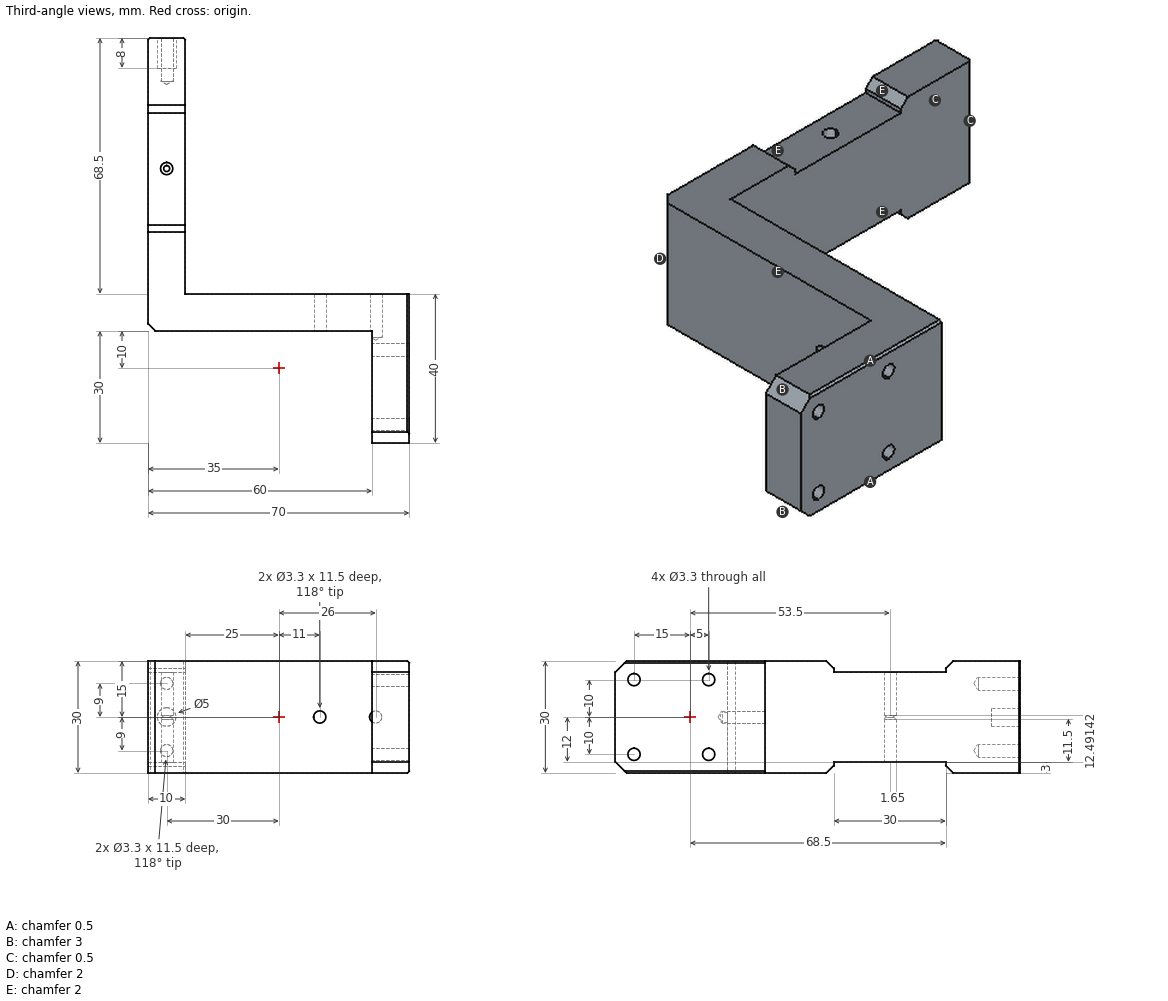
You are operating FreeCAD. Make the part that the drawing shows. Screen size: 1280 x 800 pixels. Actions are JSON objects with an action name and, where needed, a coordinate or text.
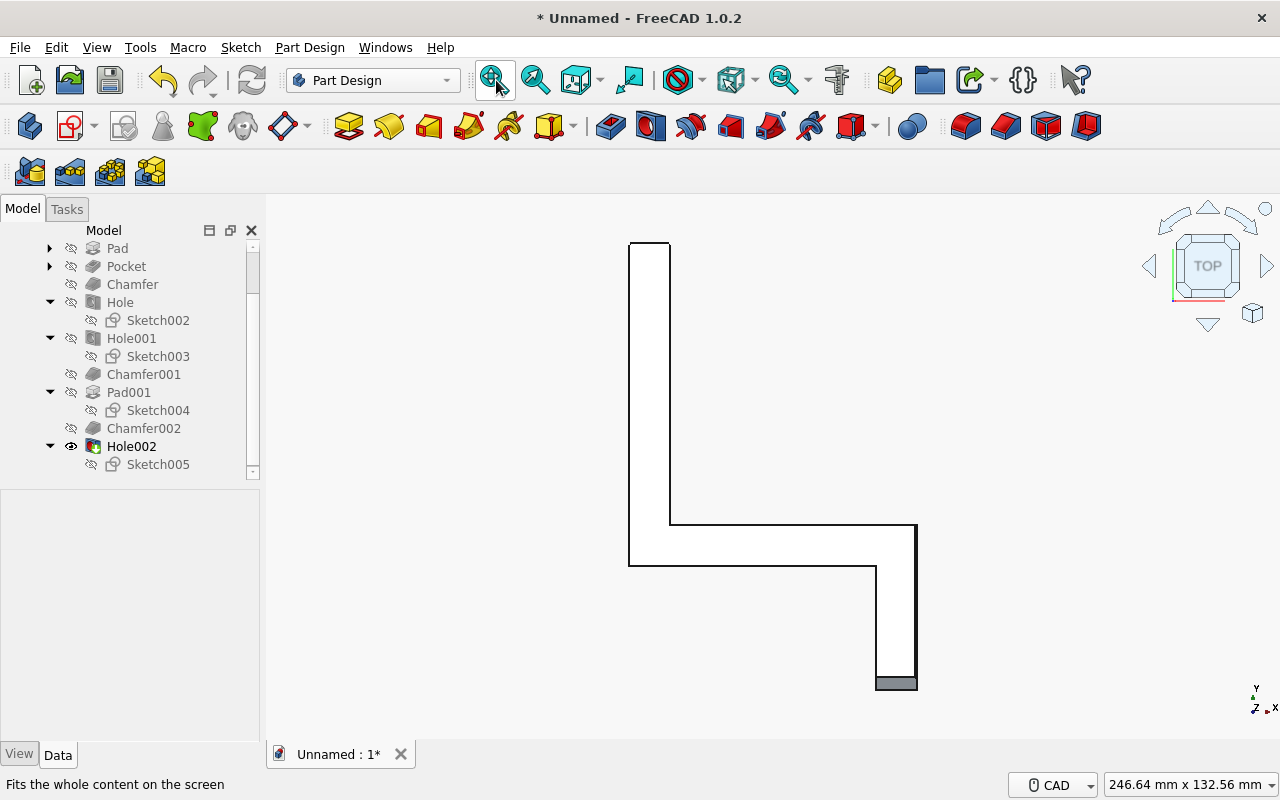
{"action": "key", "text": "1"}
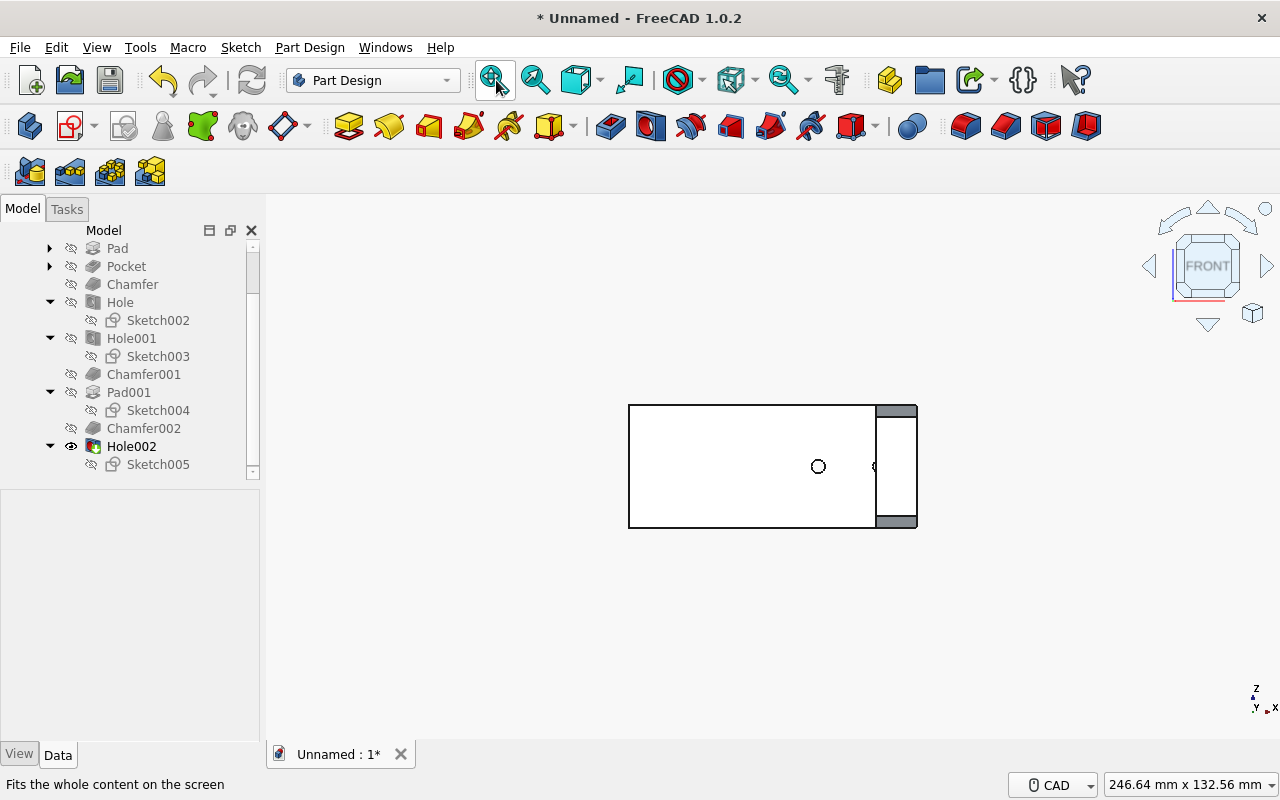
{"action": "left_click", "coordinate": [496, 80]}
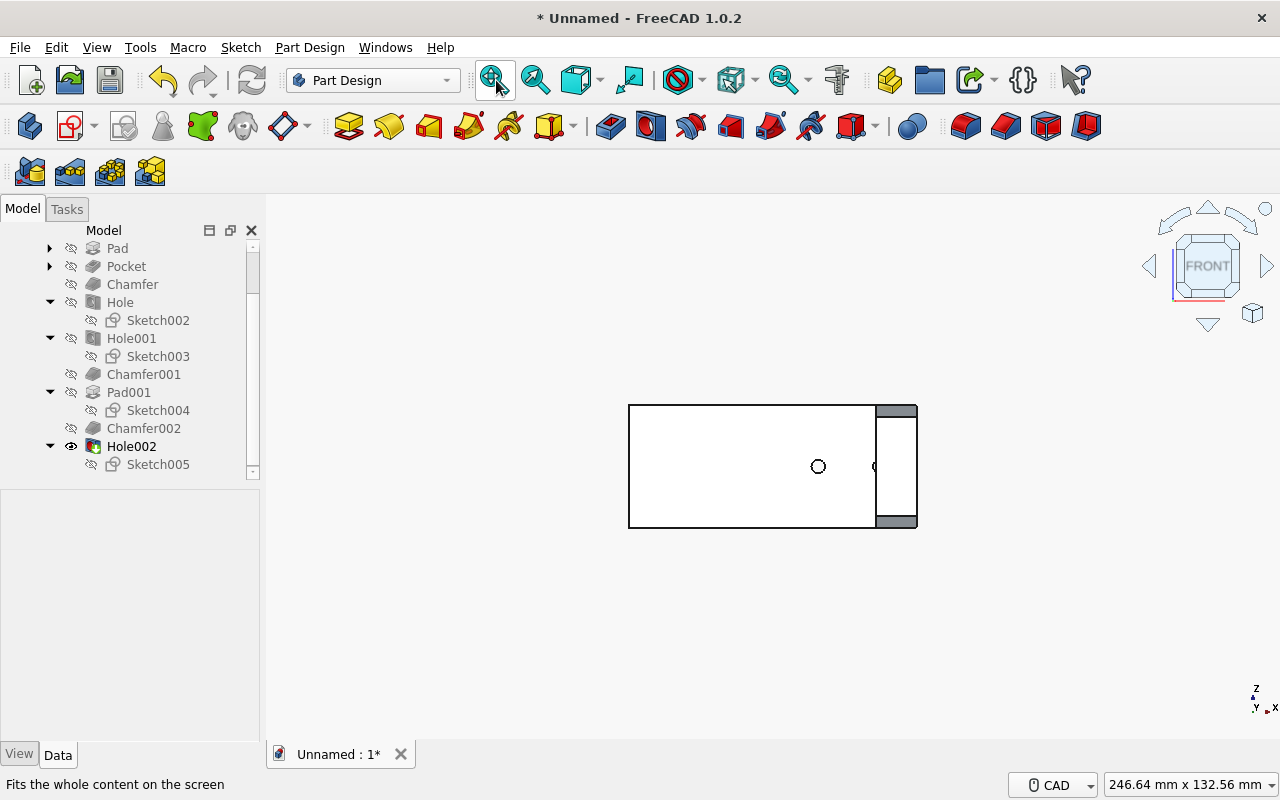
{"action": "left_click", "coordinate": [629, 466]}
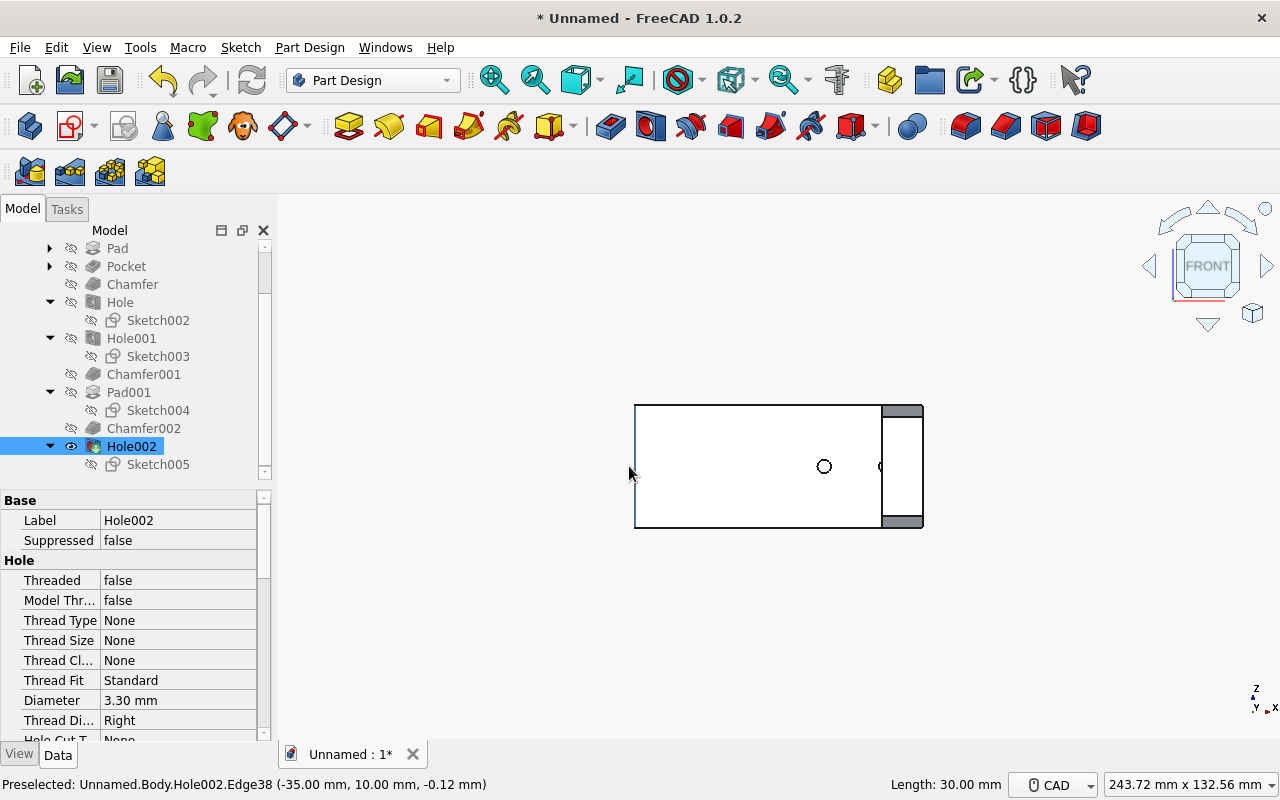
{"action": "left_click", "coordinate": [1006, 126]}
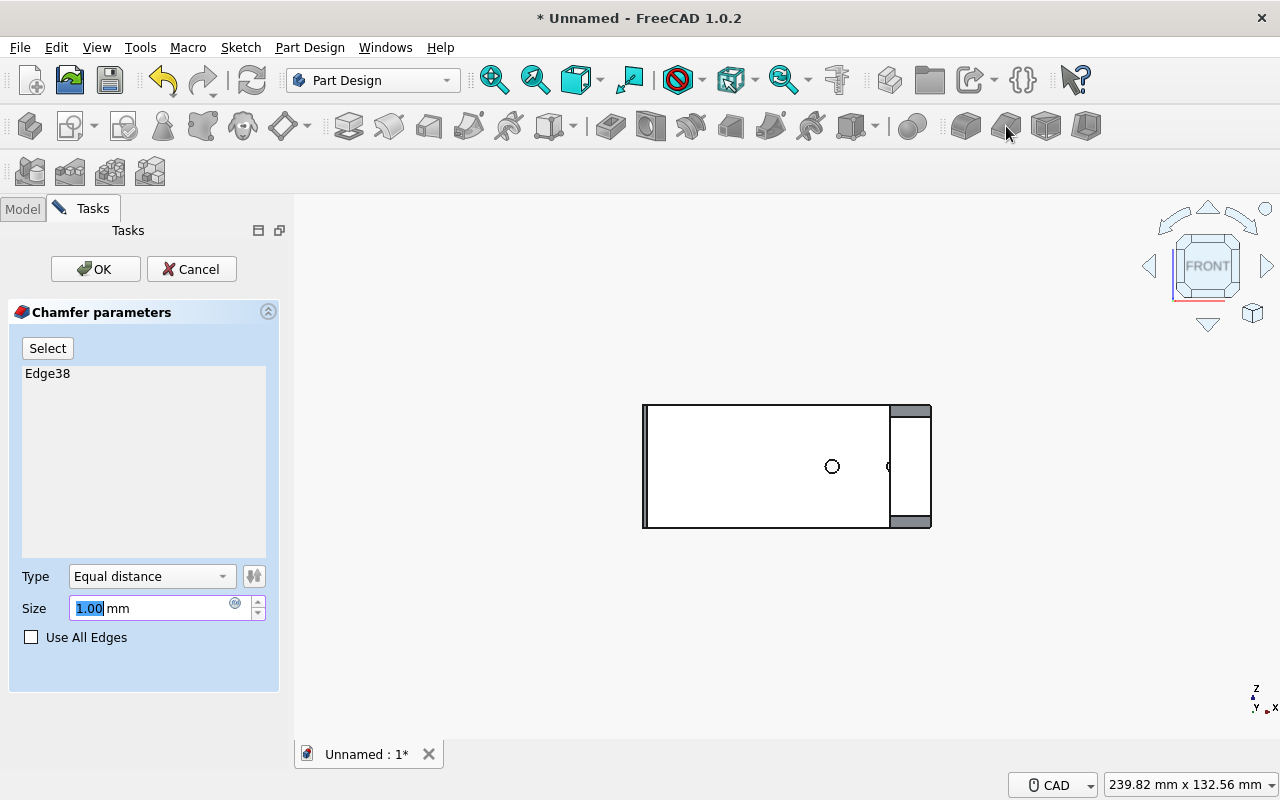
{"action": "type", "text": "2"}
{"action": "key", "text": "Tab"}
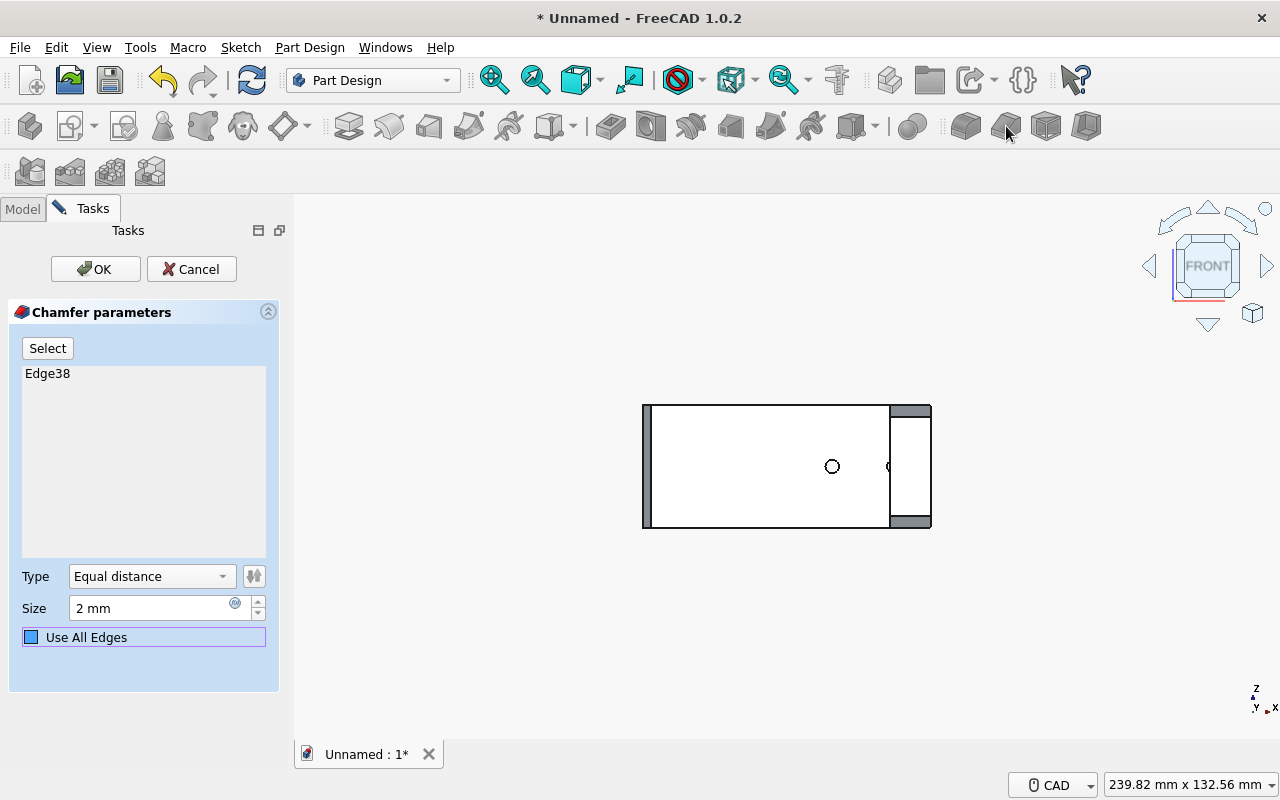
{"action": "left_click", "coordinate": [96, 269]}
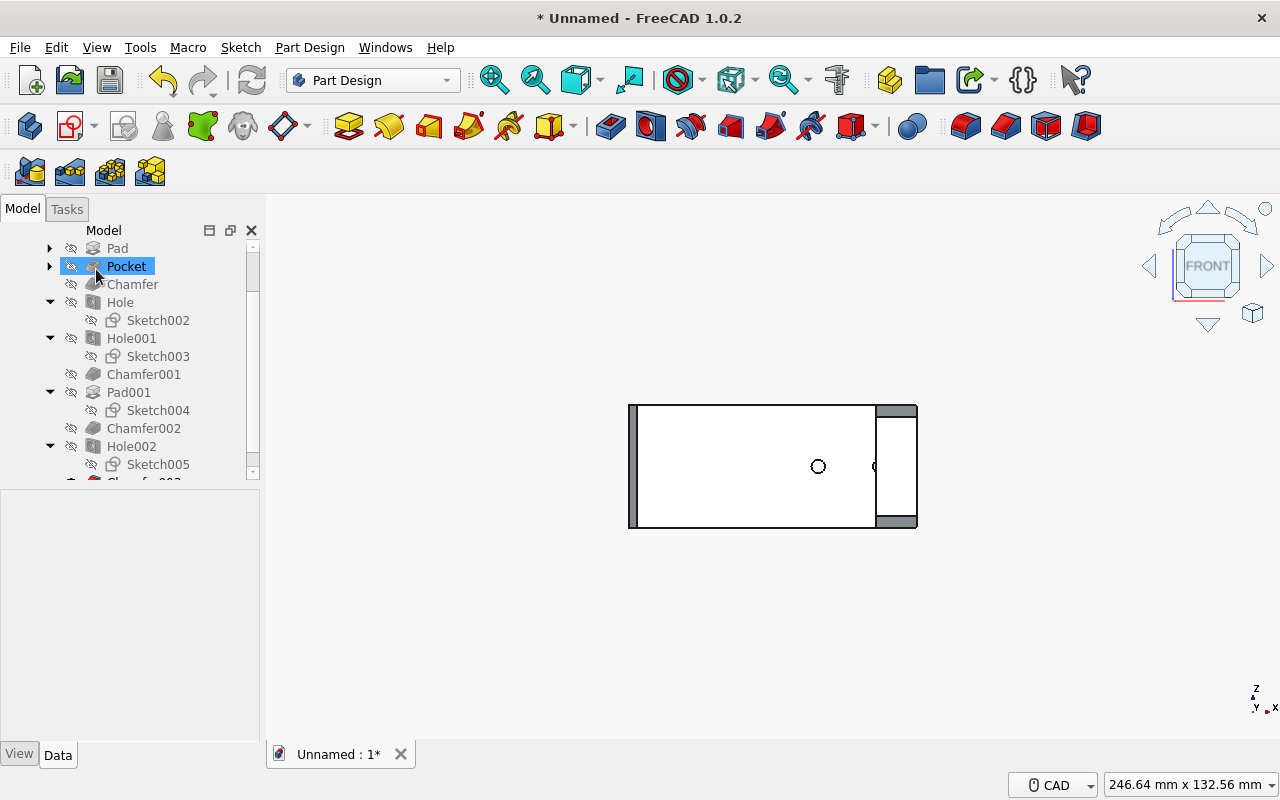
{"action": "left_click", "coordinate": [496, 80]}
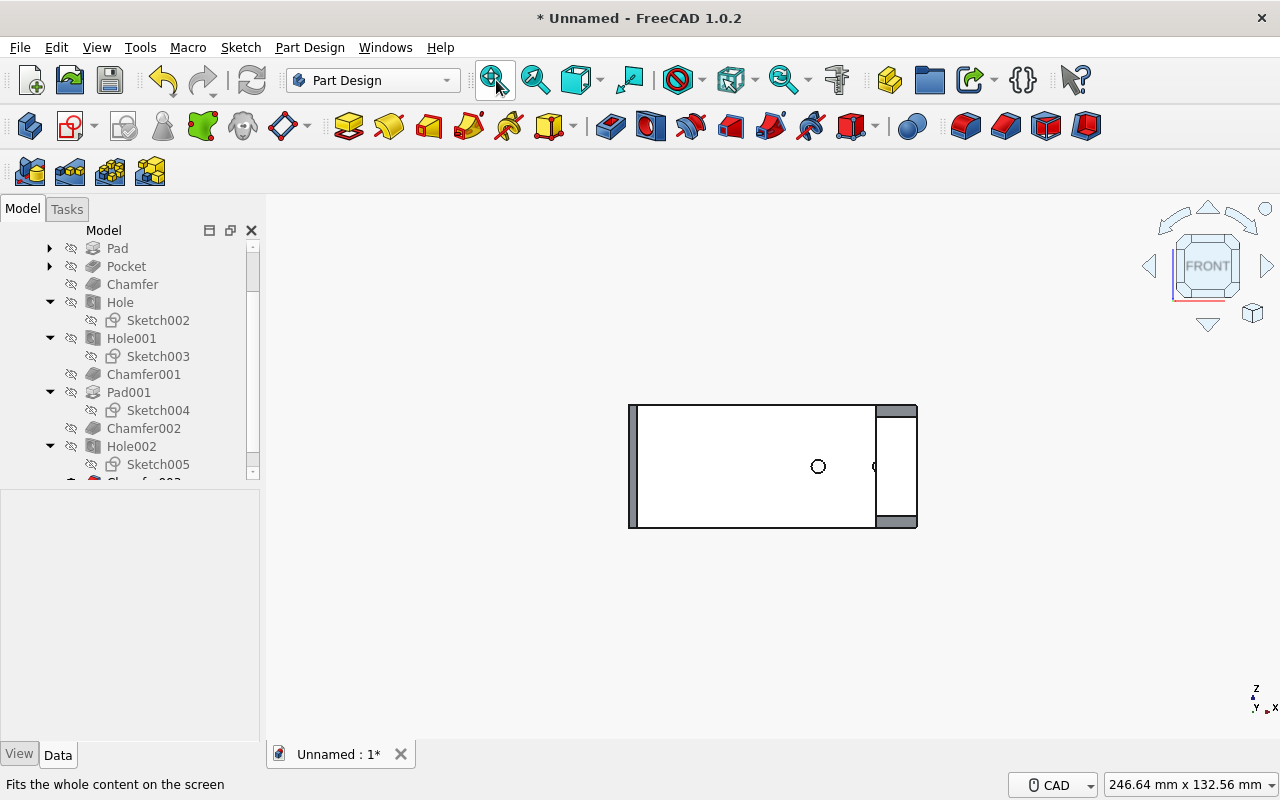
{"action": "key", "text": "4"}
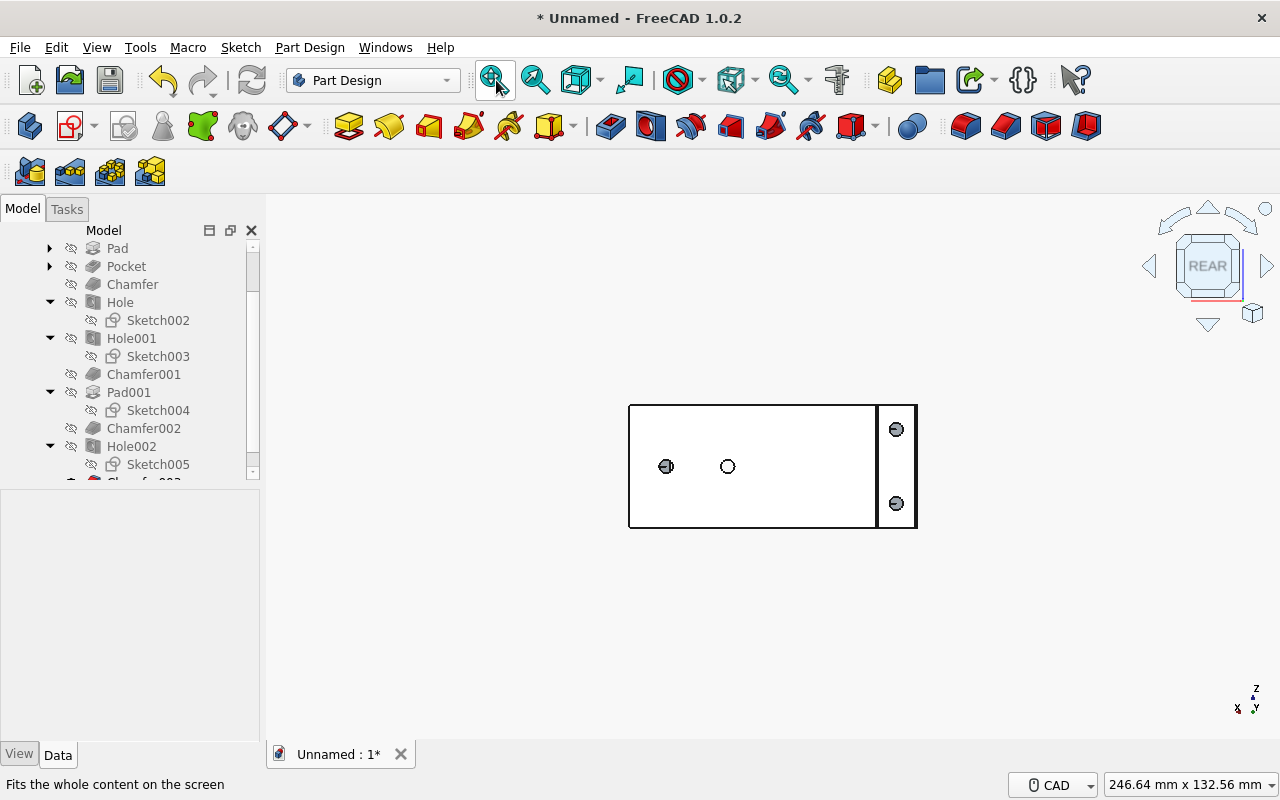
{"action": "key", "text": "v f"}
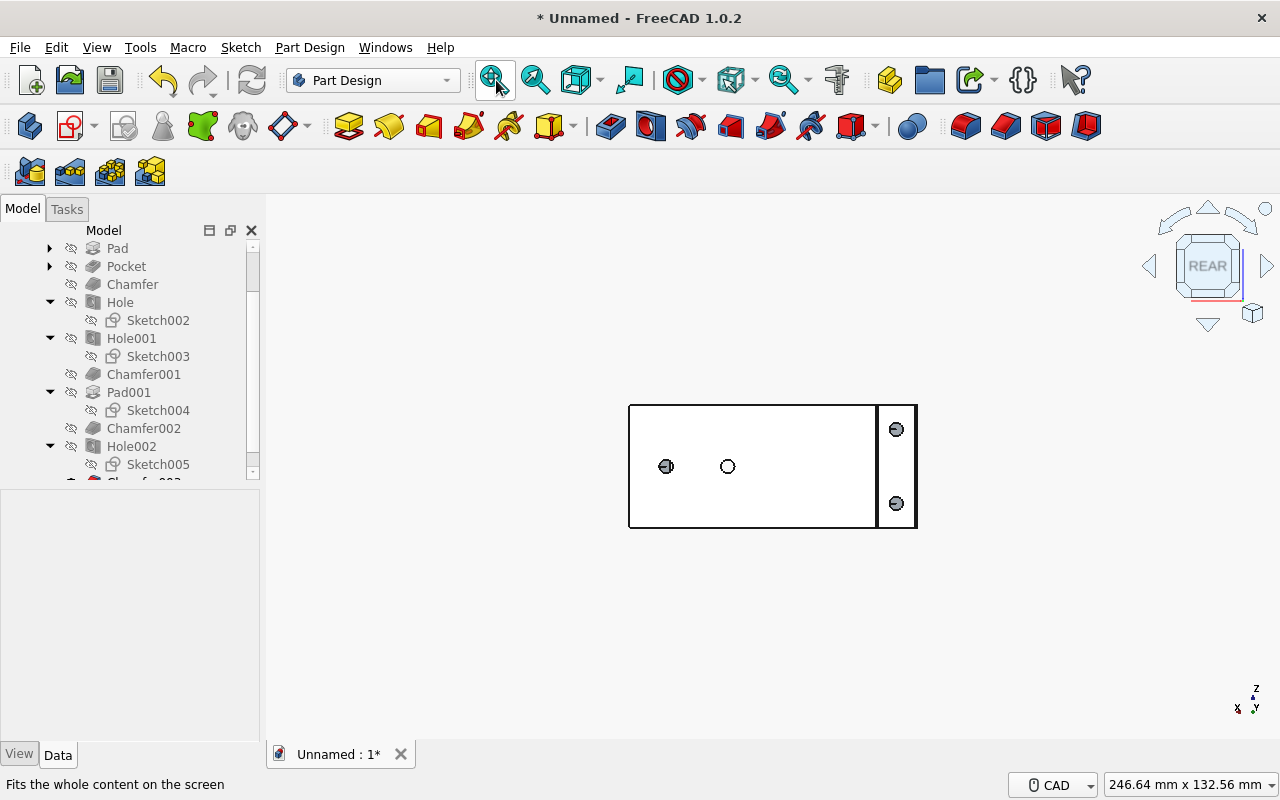
{"action": "left_click", "coordinate": [896, 466]}